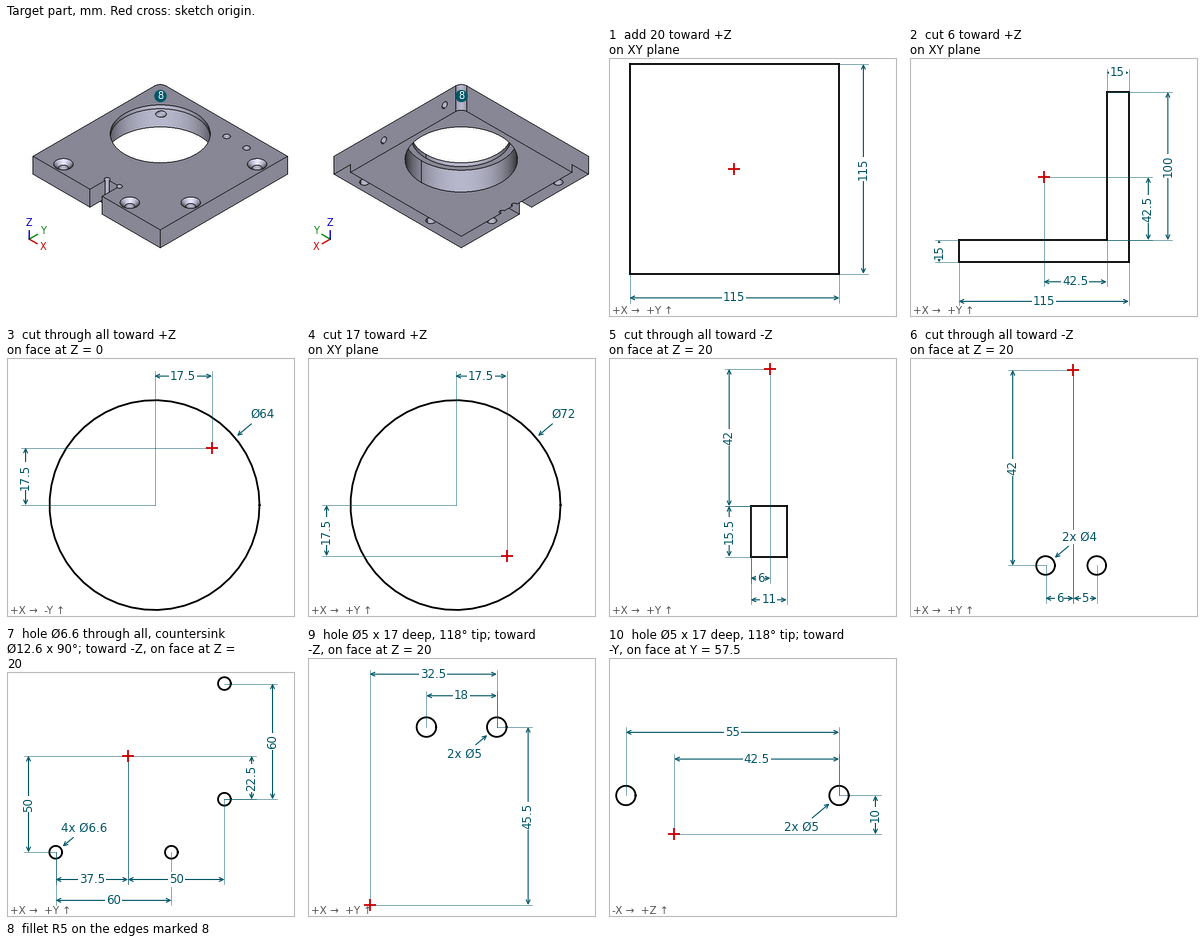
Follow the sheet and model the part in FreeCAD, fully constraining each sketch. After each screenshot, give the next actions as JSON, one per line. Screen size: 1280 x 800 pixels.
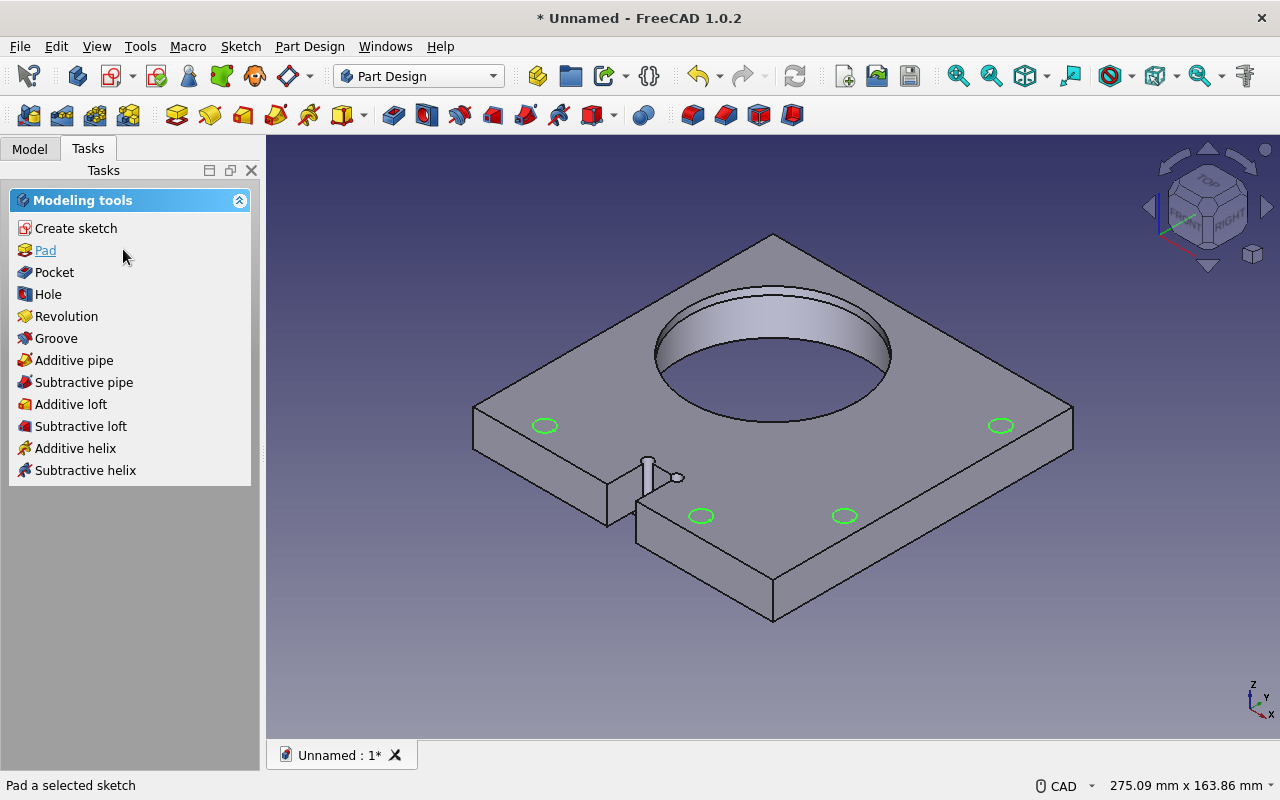
{"action": "left_click", "coordinate": [427, 116]}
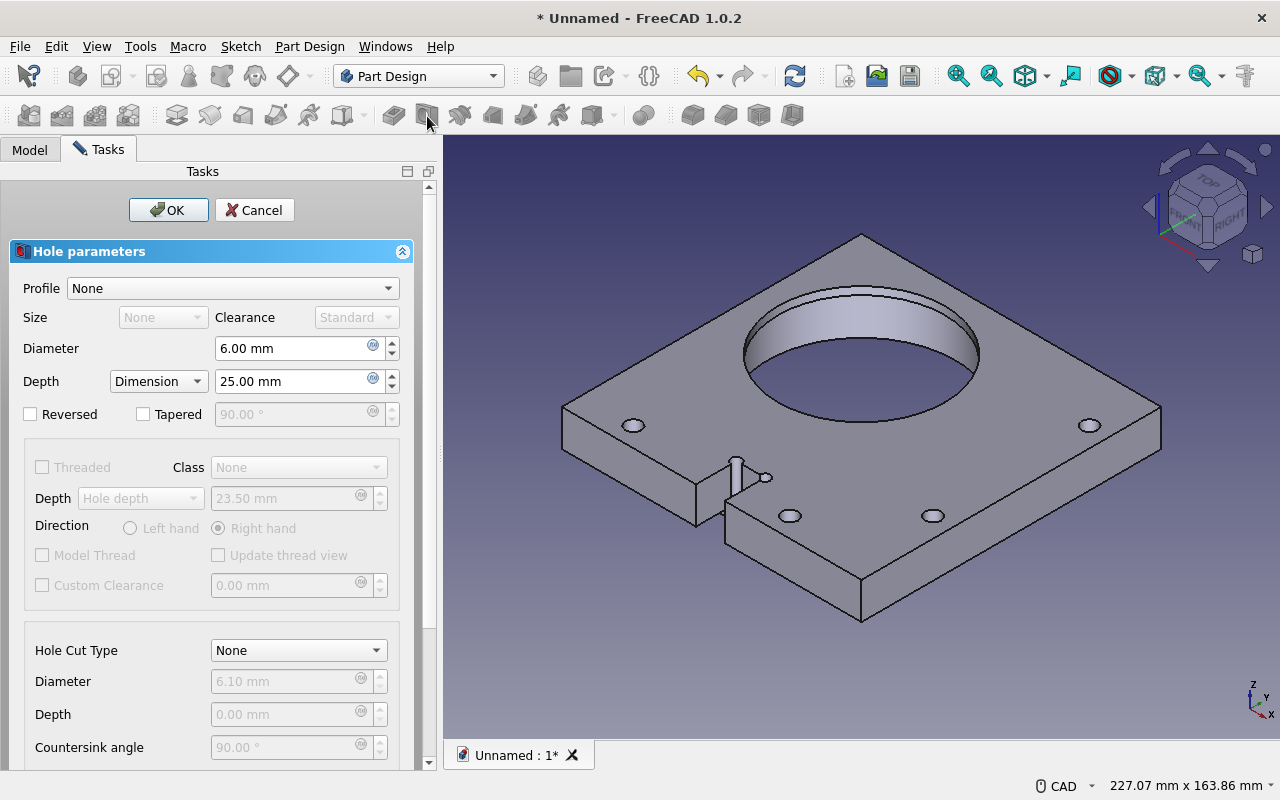
{"action": "triple_click", "coordinate": [300, 348]}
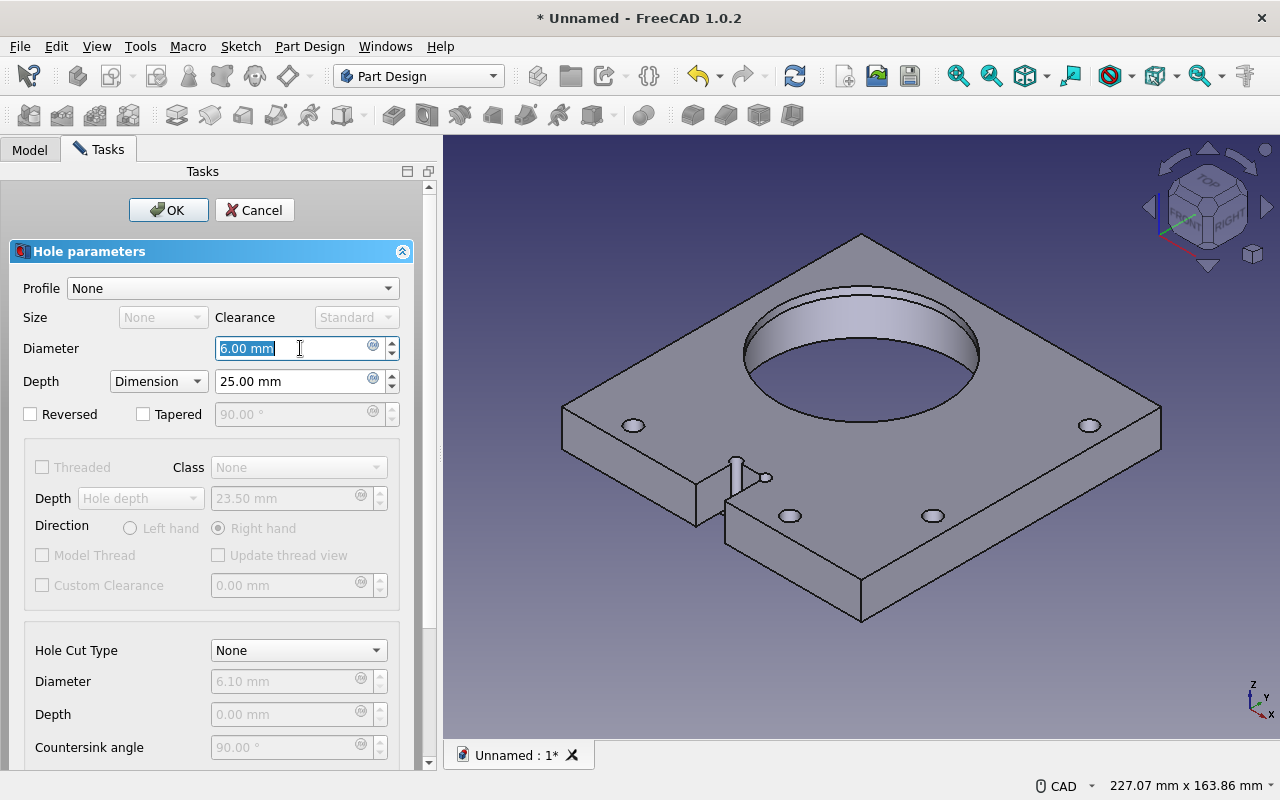
{"action": "type", "text": "6.6"}
{"action": "key", "text": "Tab"}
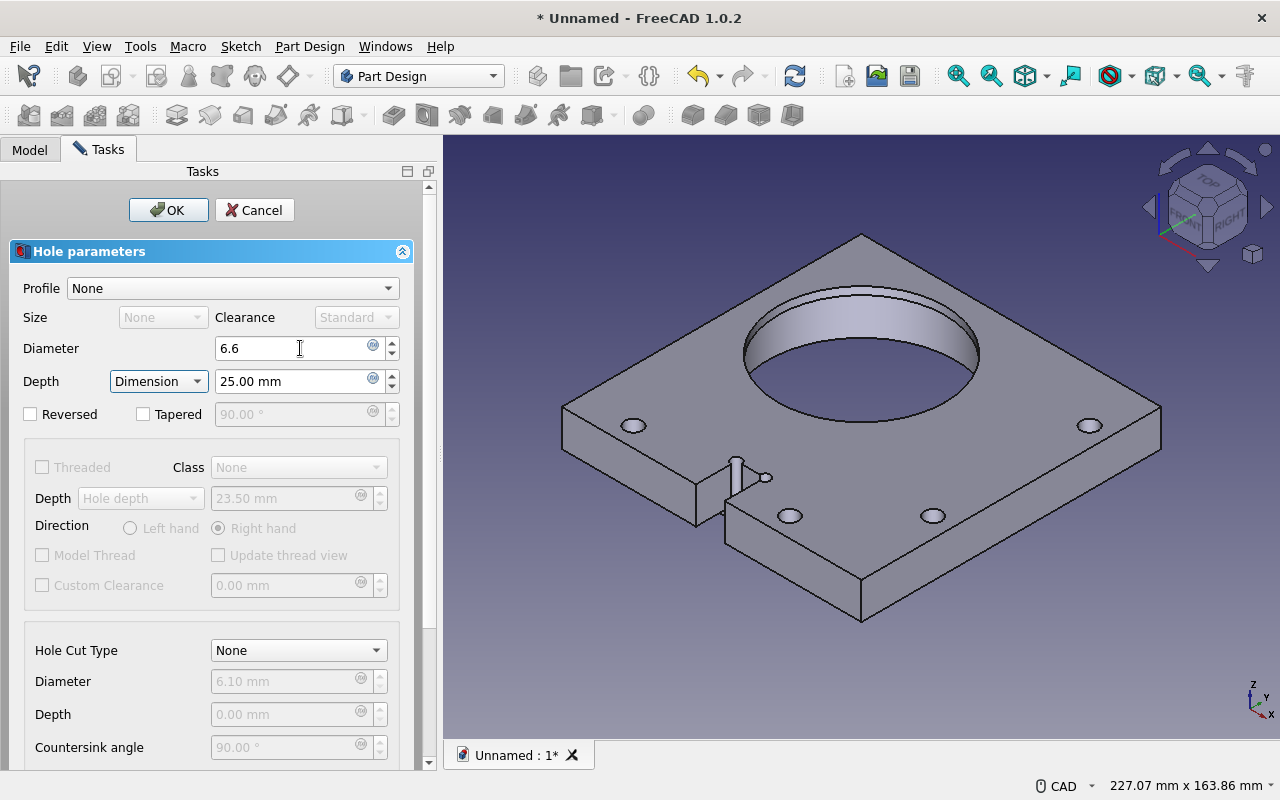
{"action": "left_click", "coordinate": [160, 382]}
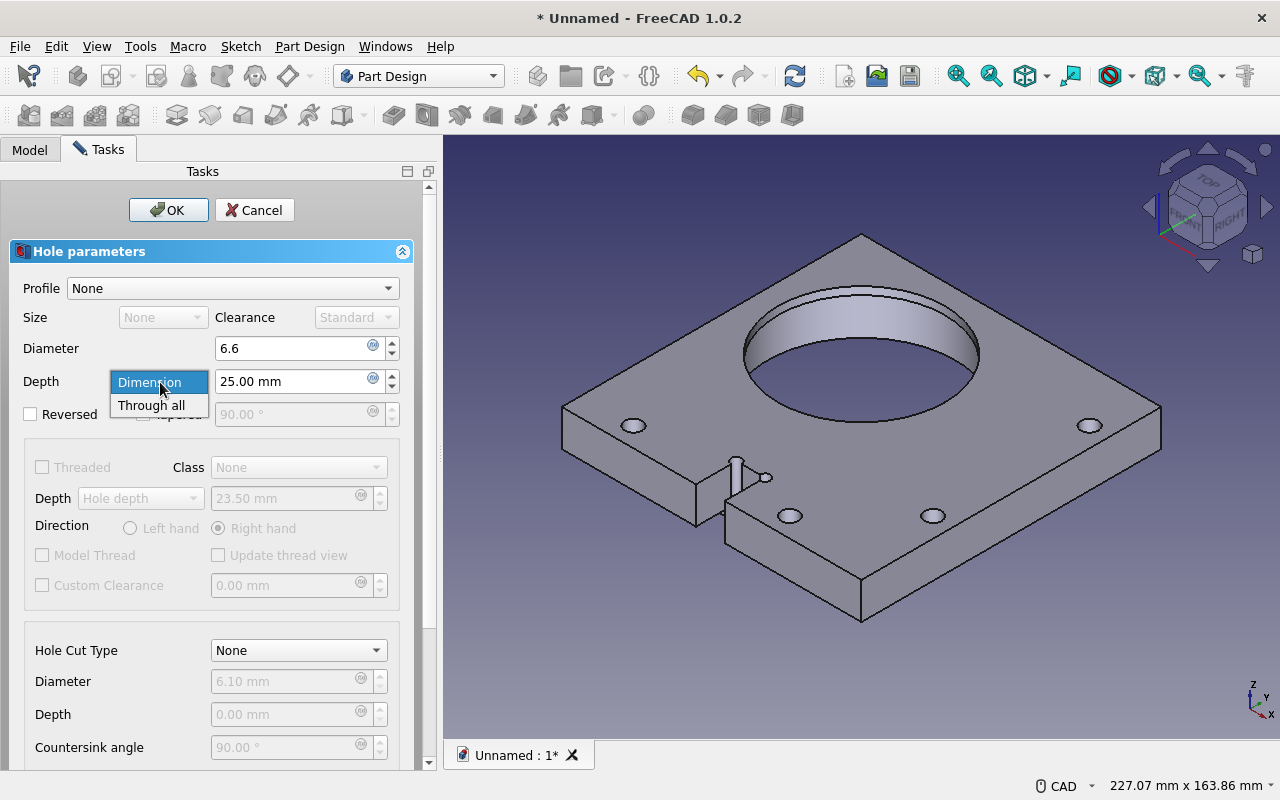
{"action": "left_click", "coordinate": [158, 406]}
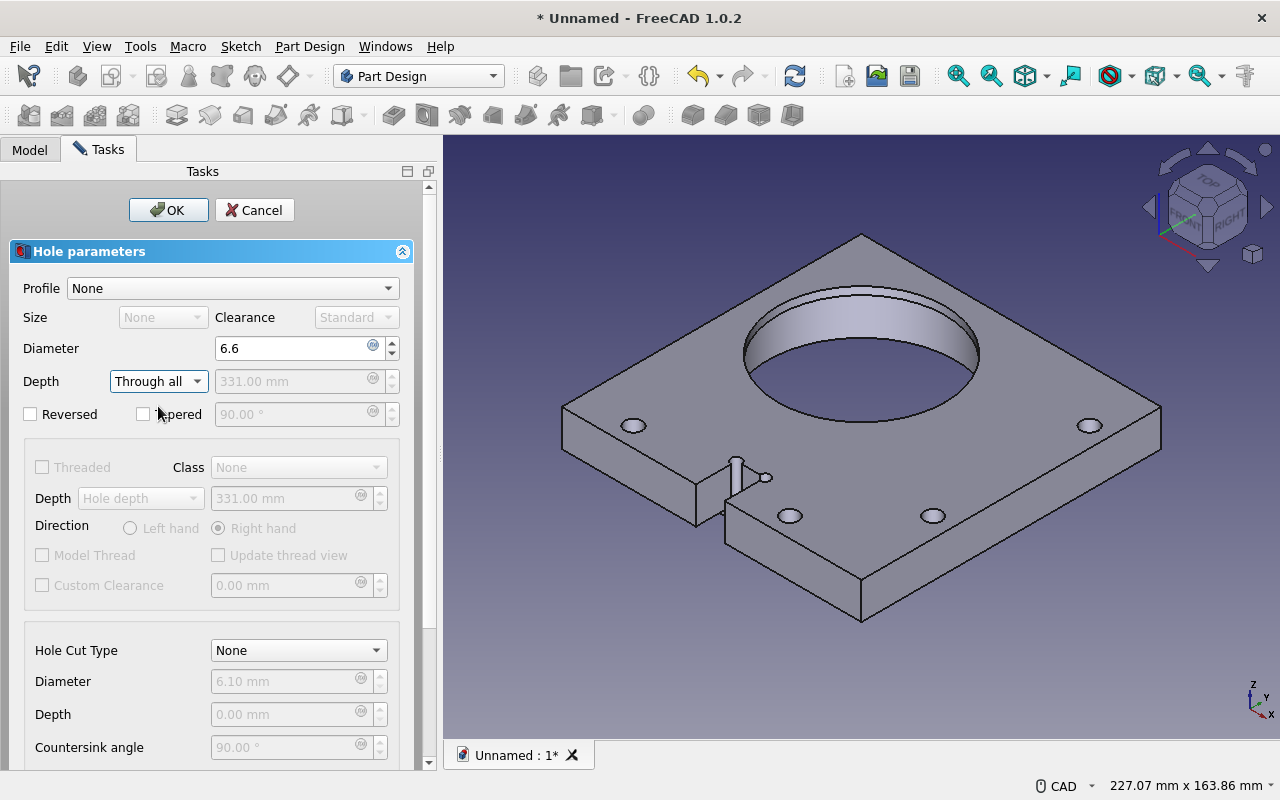
{"action": "left_click", "coordinate": [300, 650]}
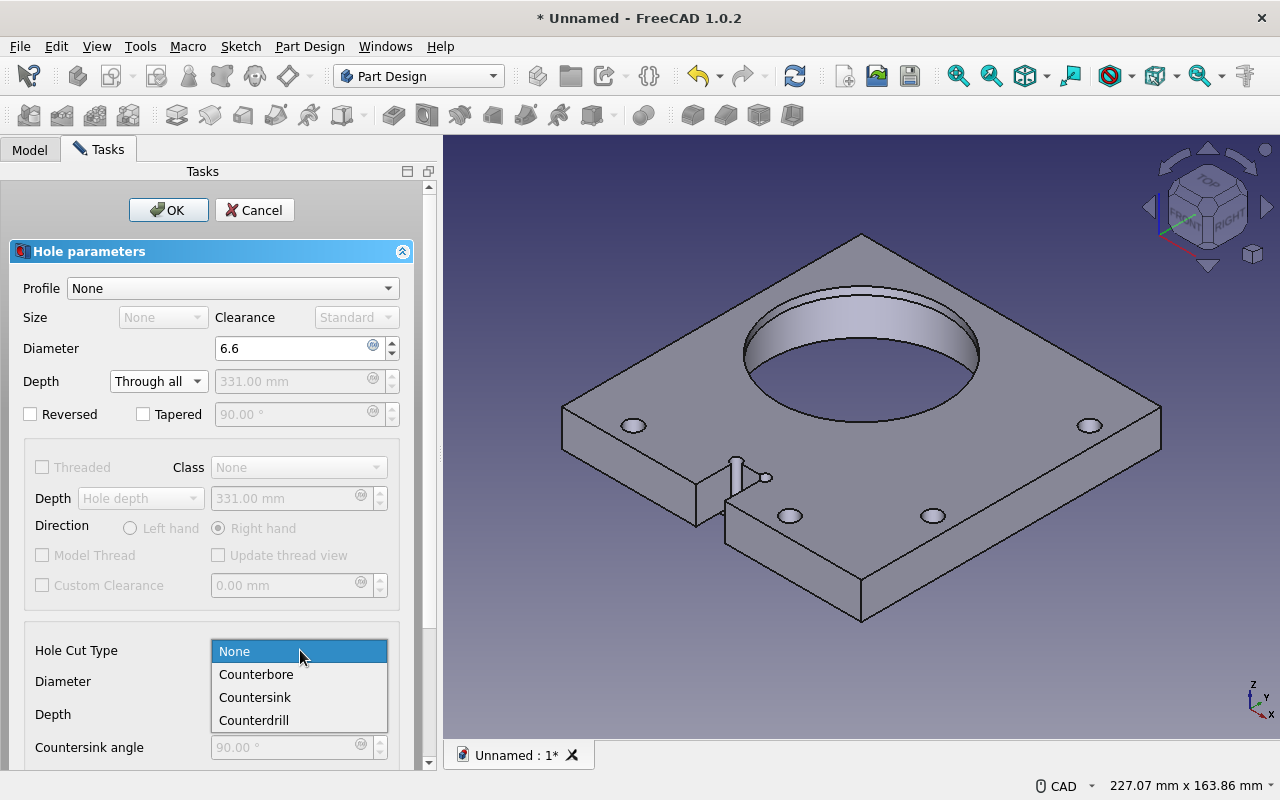
{"action": "left_click", "coordinate": [298, 698]}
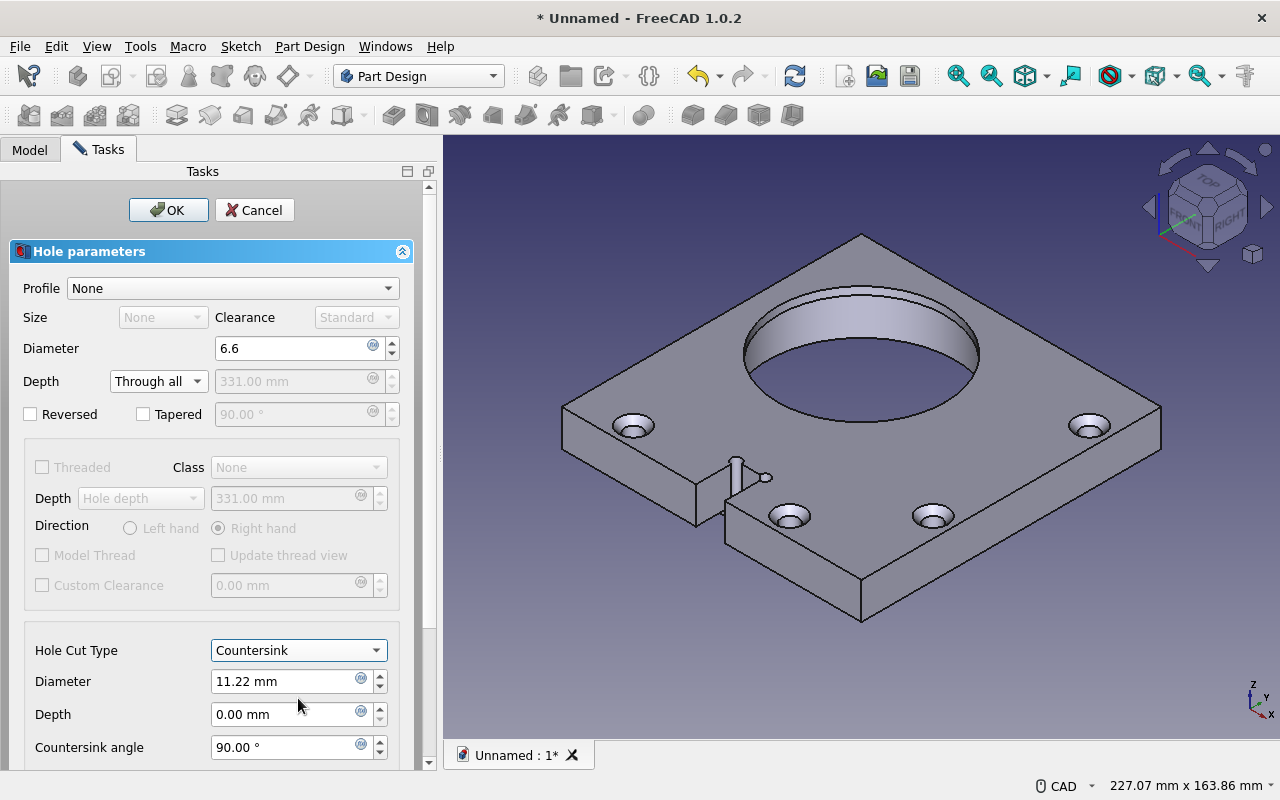
{"action": "triple_click", "coordinate": [292, 682]}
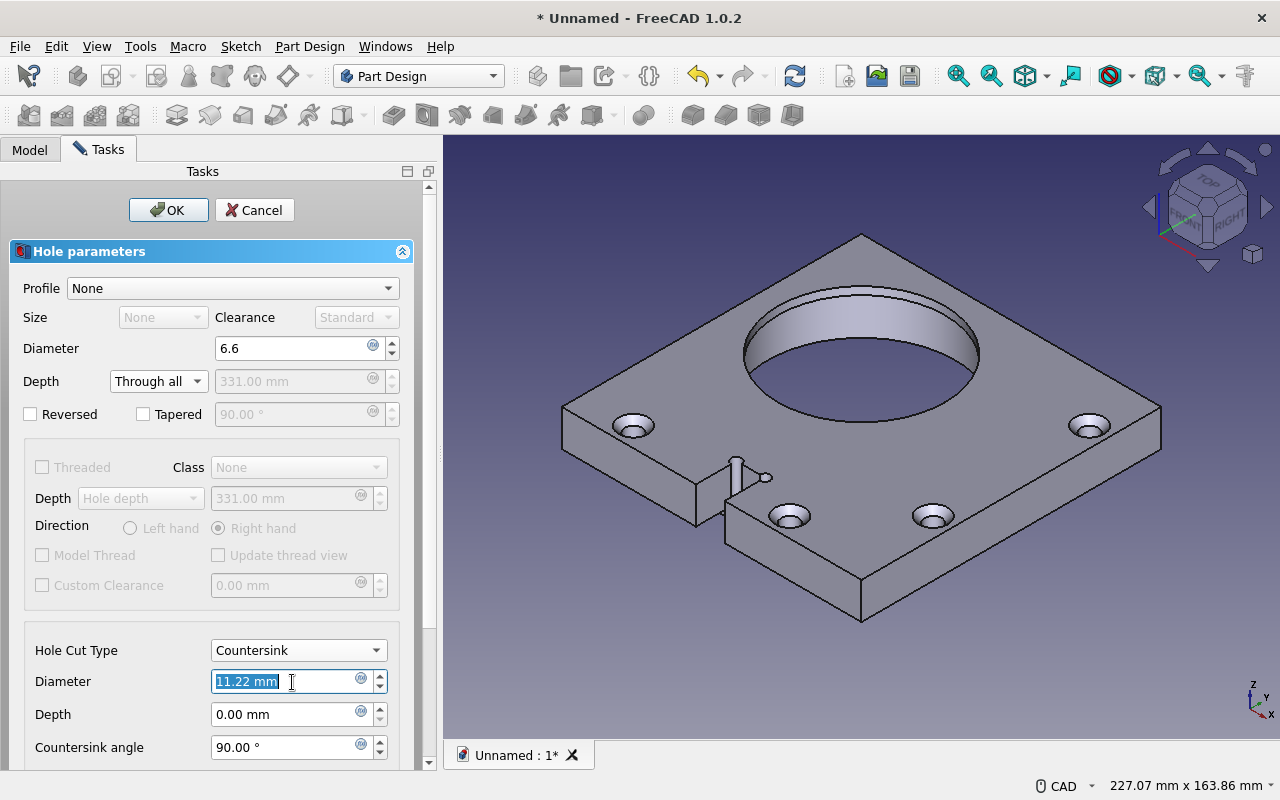
{"action": "type", "text": "12.6"}
{"action": "key", "text": "Tab"}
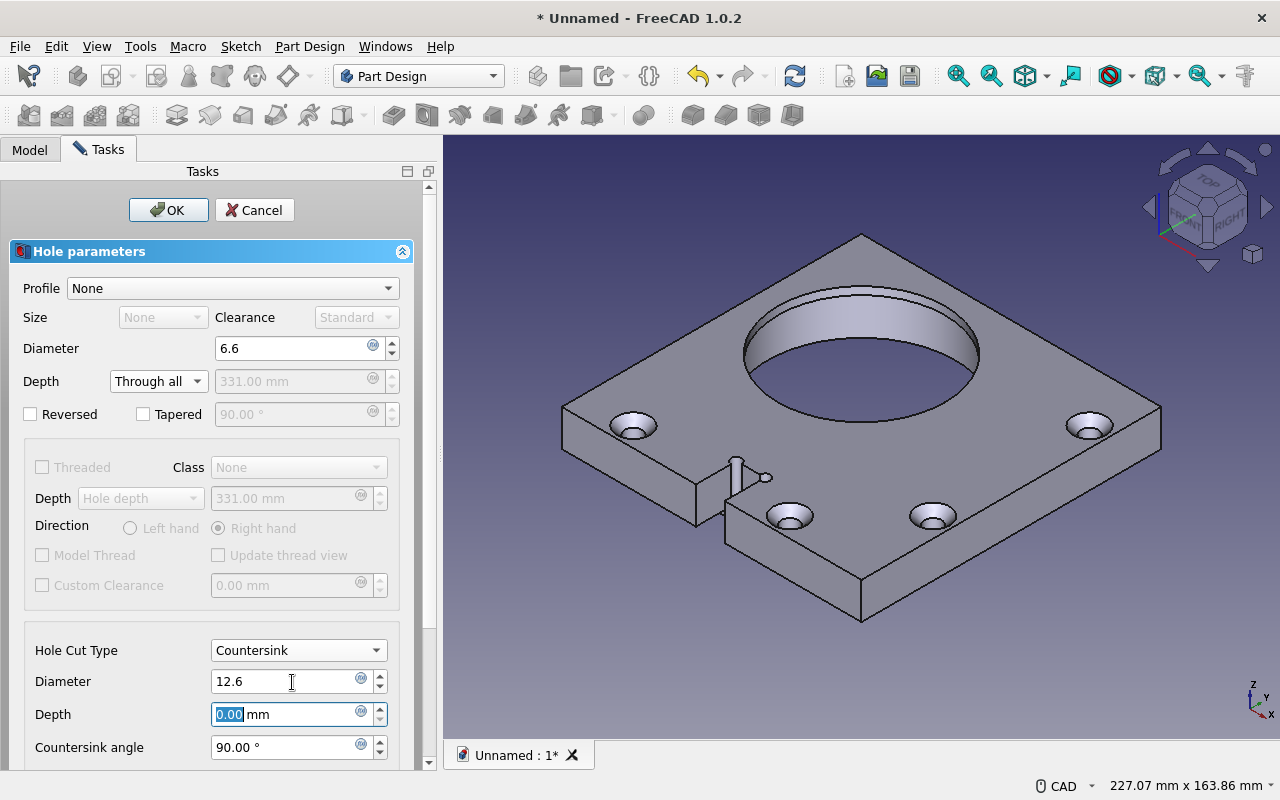
{"action": "left_click", "coordinate": [169, 210]}